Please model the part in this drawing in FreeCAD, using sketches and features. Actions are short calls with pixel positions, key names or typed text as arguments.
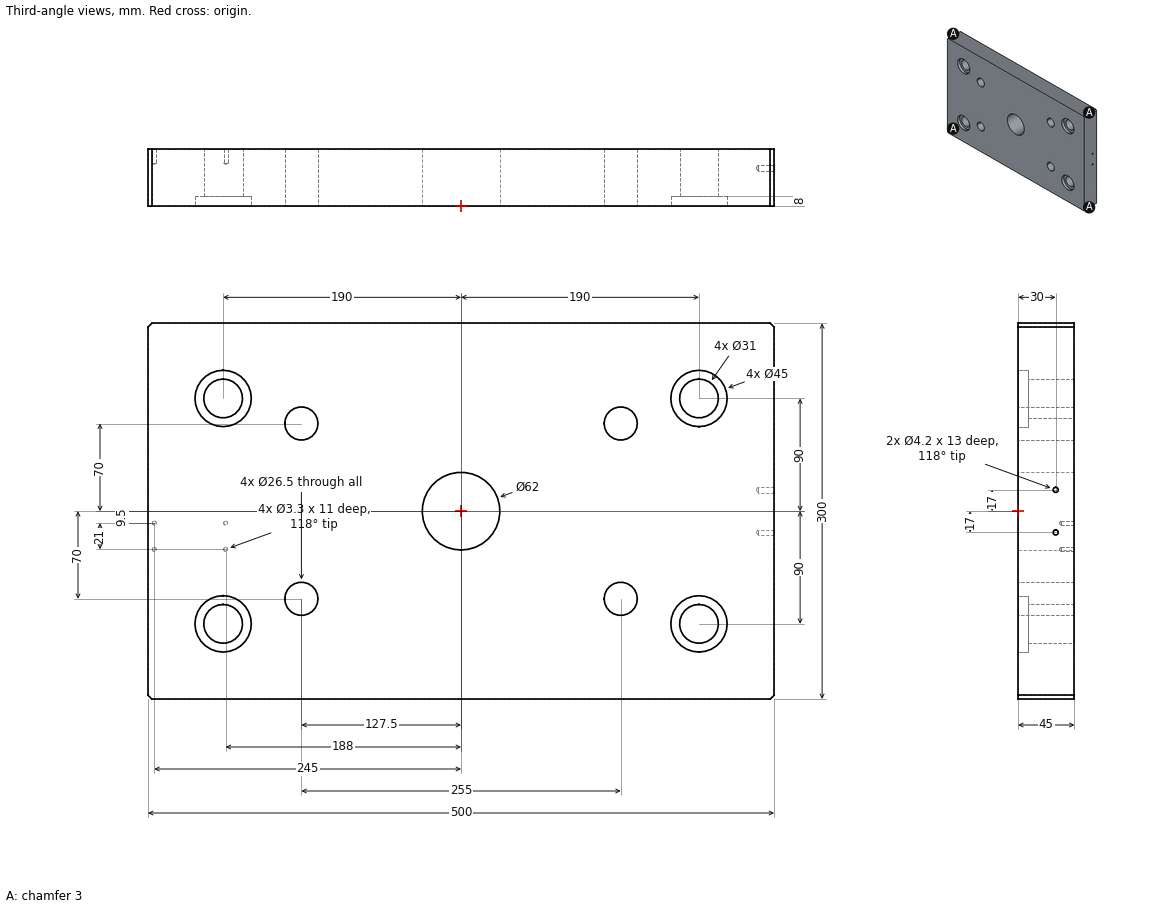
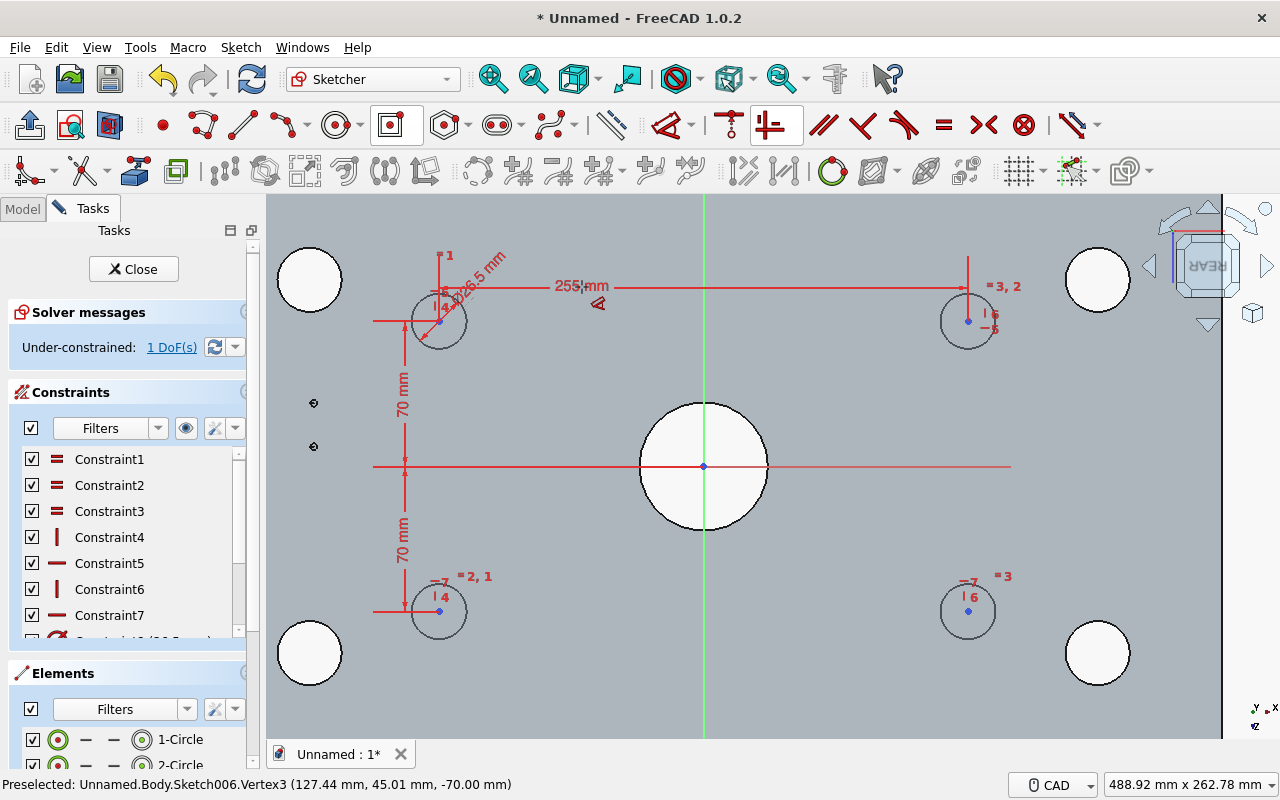
click(439, 321)
click(664, 287)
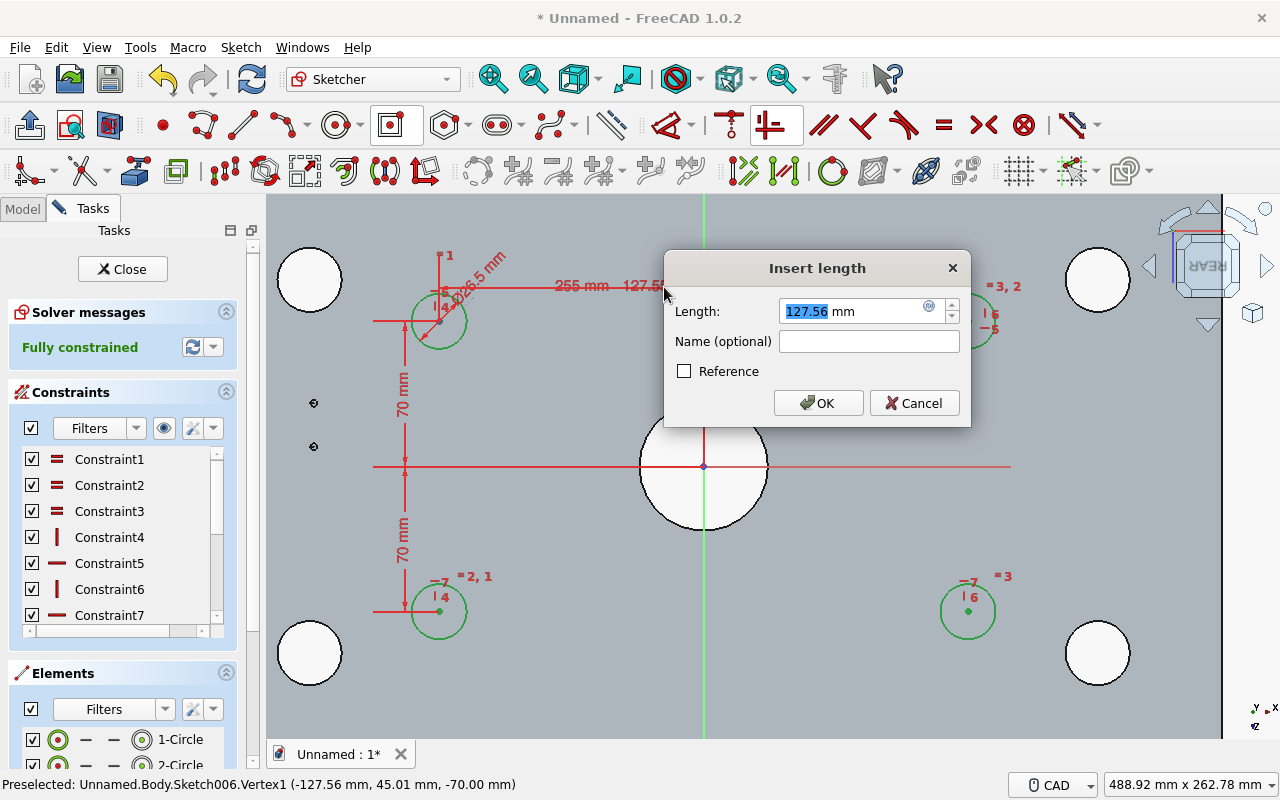
text(127.5)
key(Return)
key(Escape)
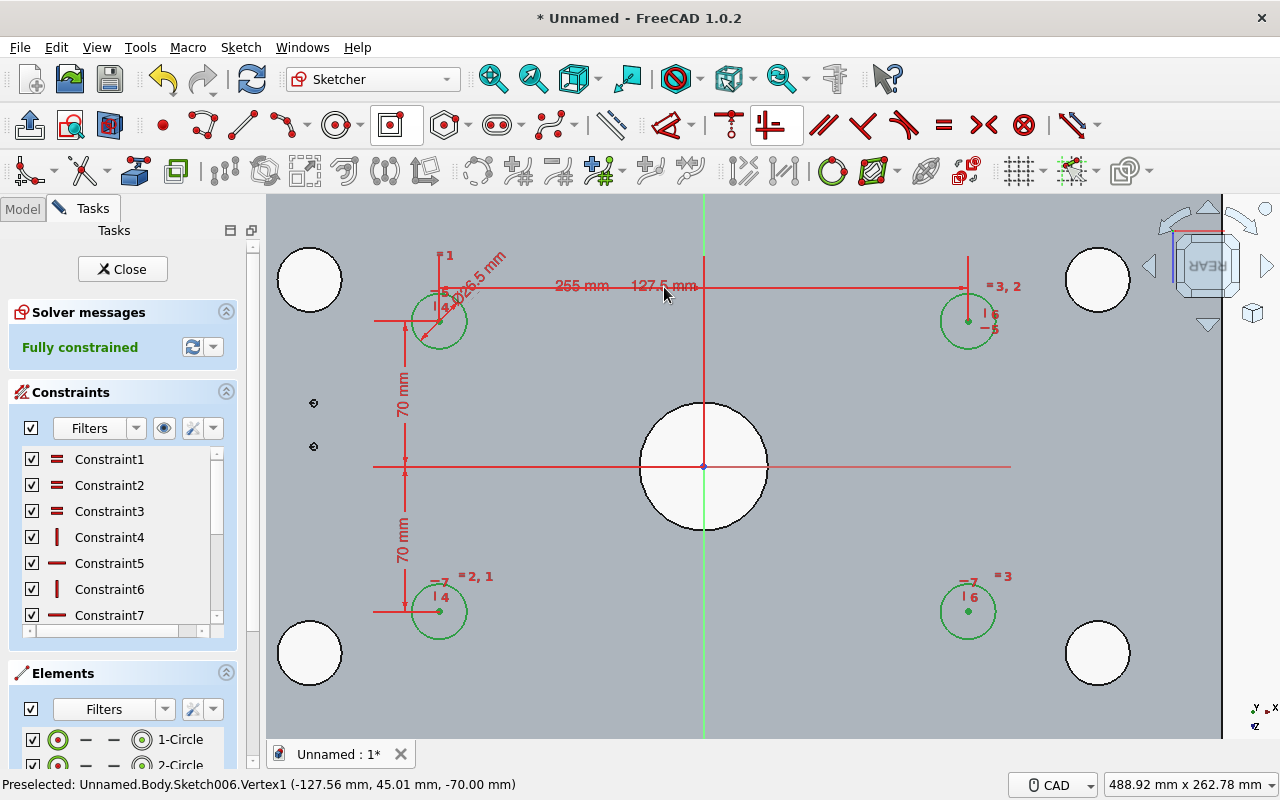
click(123, 269)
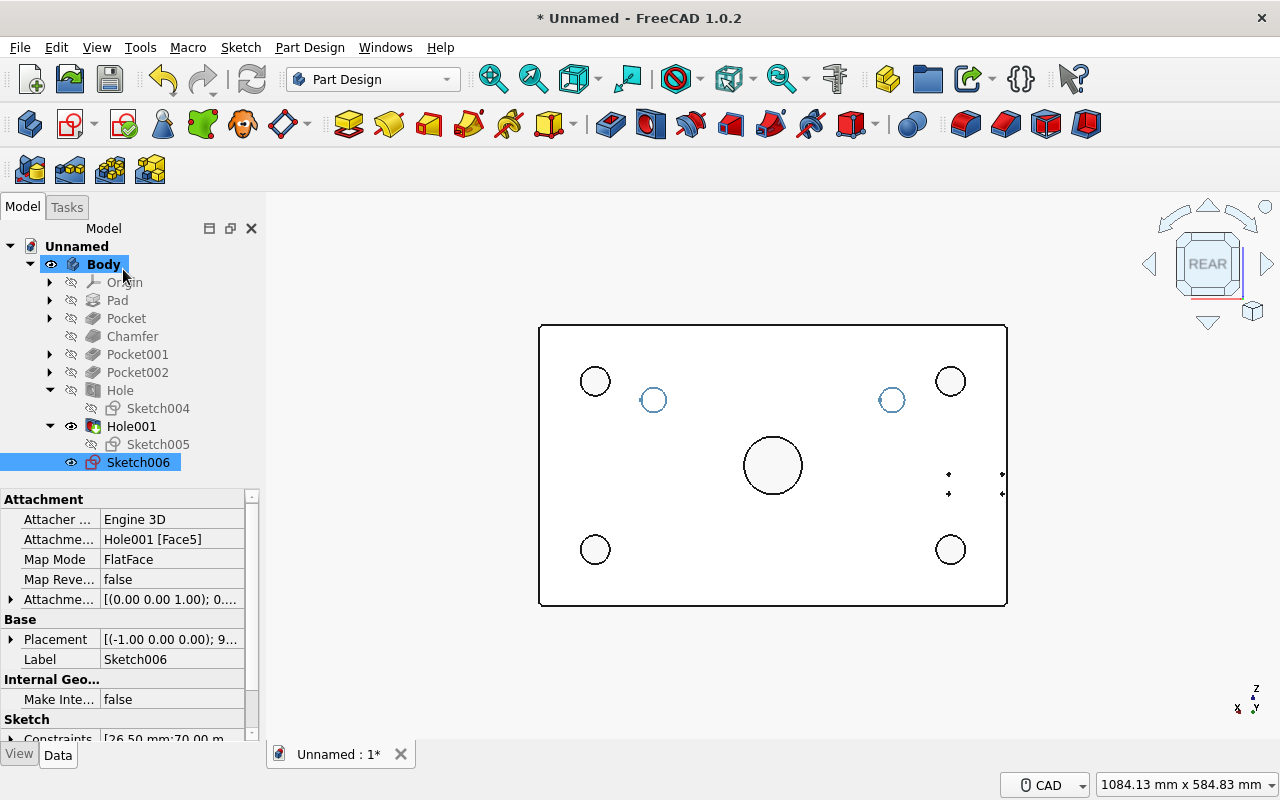
click(652, 124)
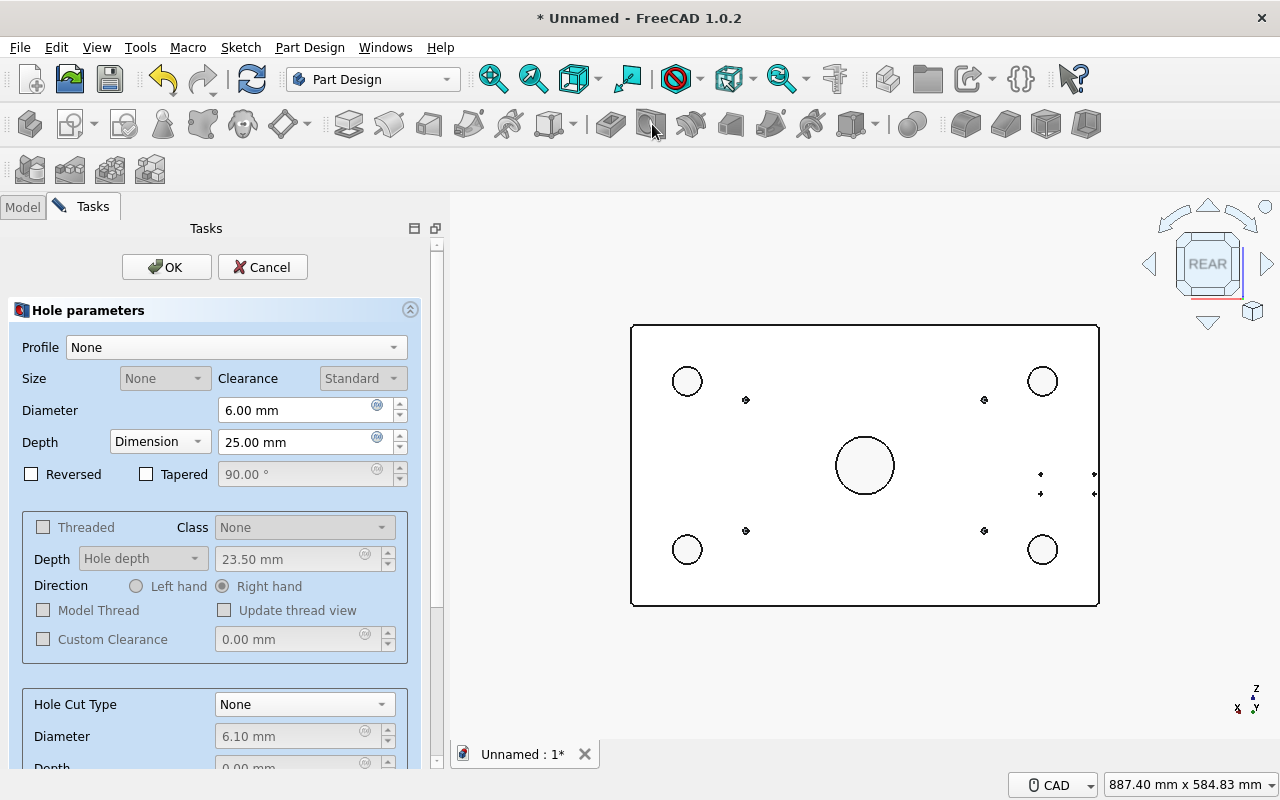
triple_click(305, 410)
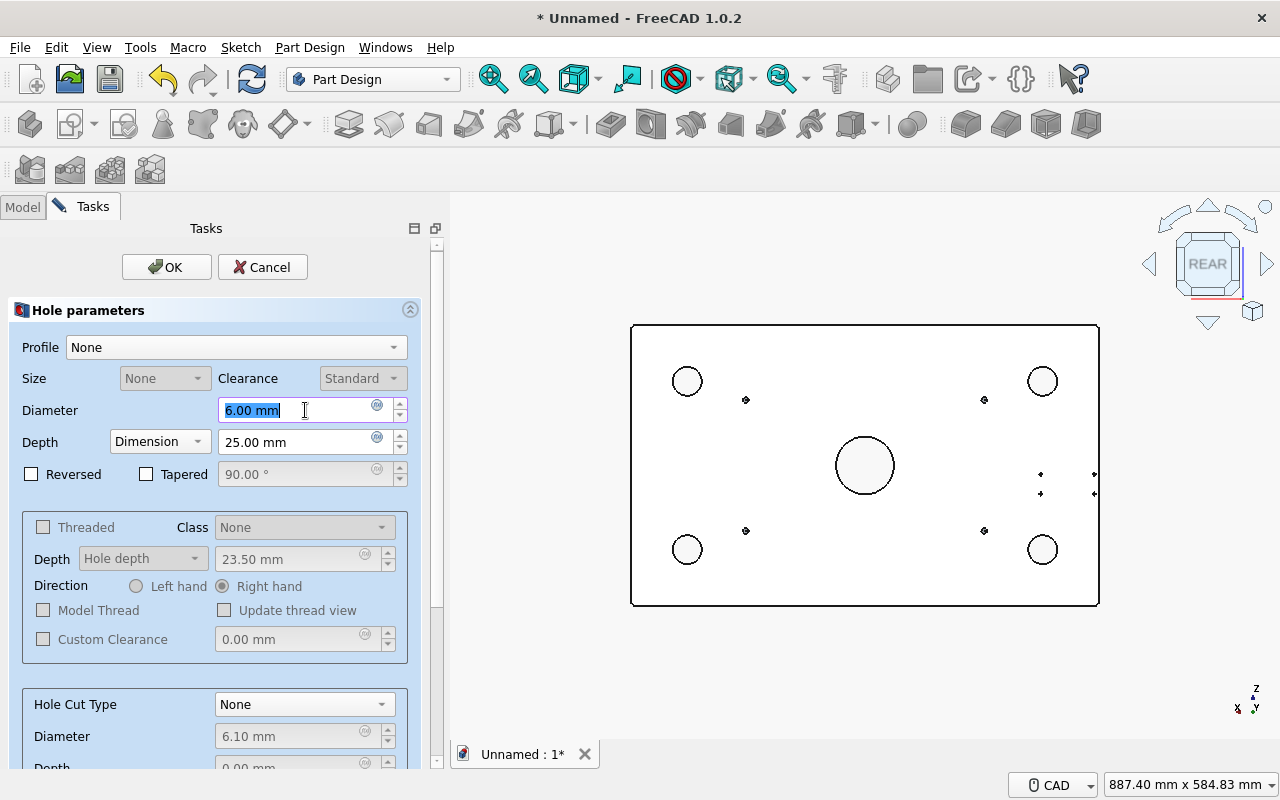
text(26.5)
key(Tab)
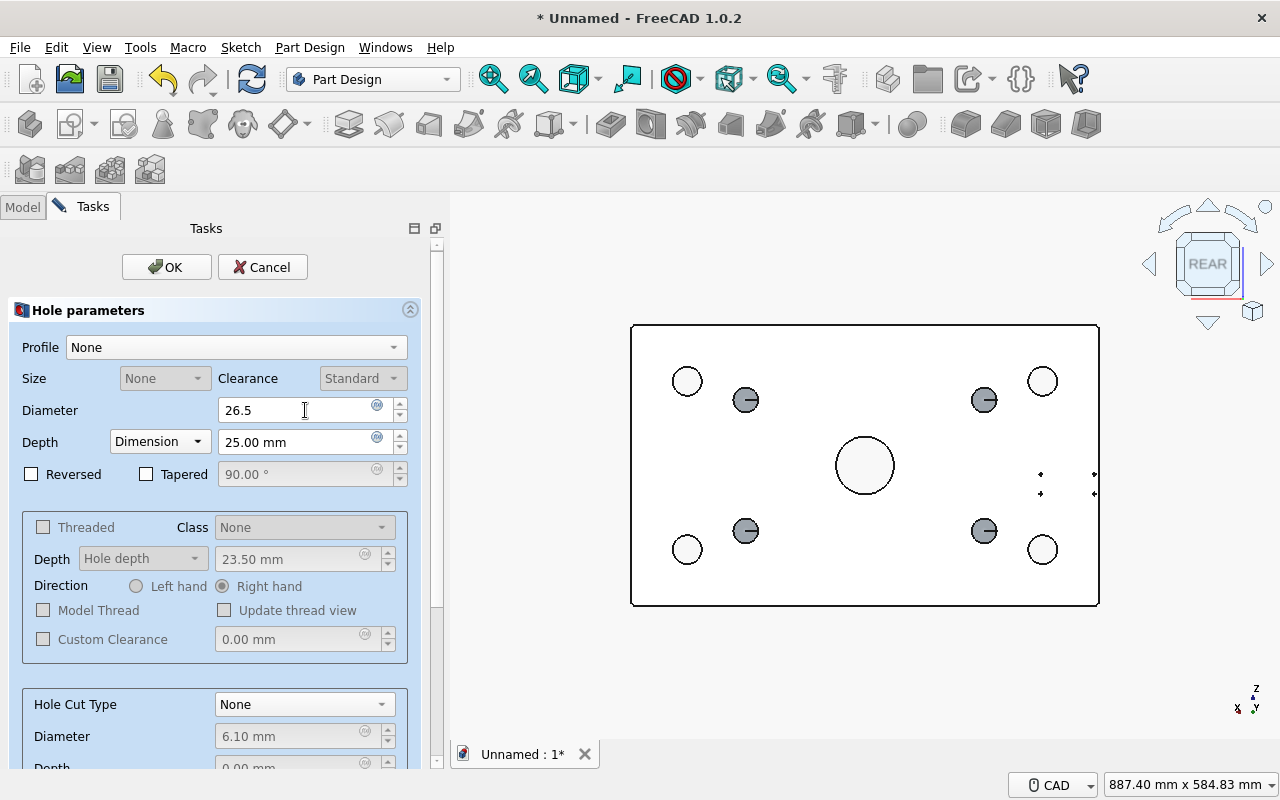
click(161, 442)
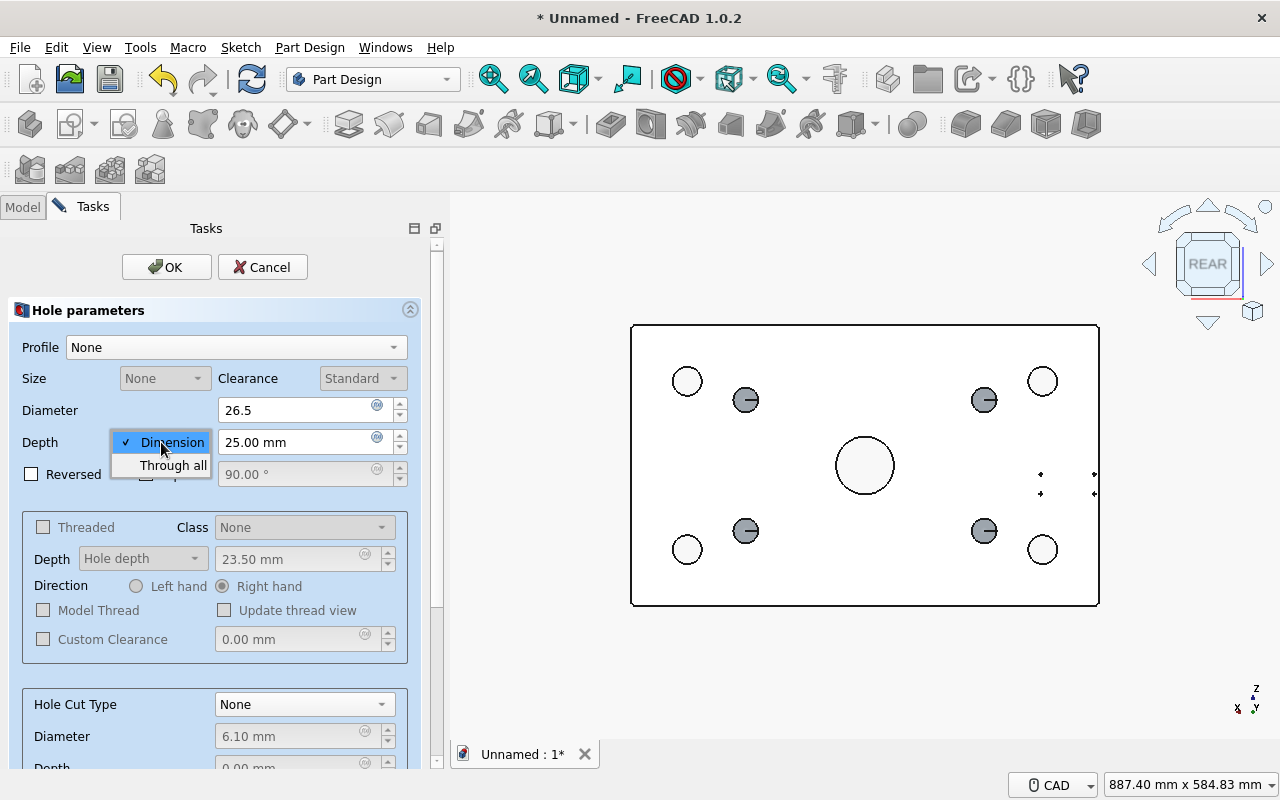
click(160, 466)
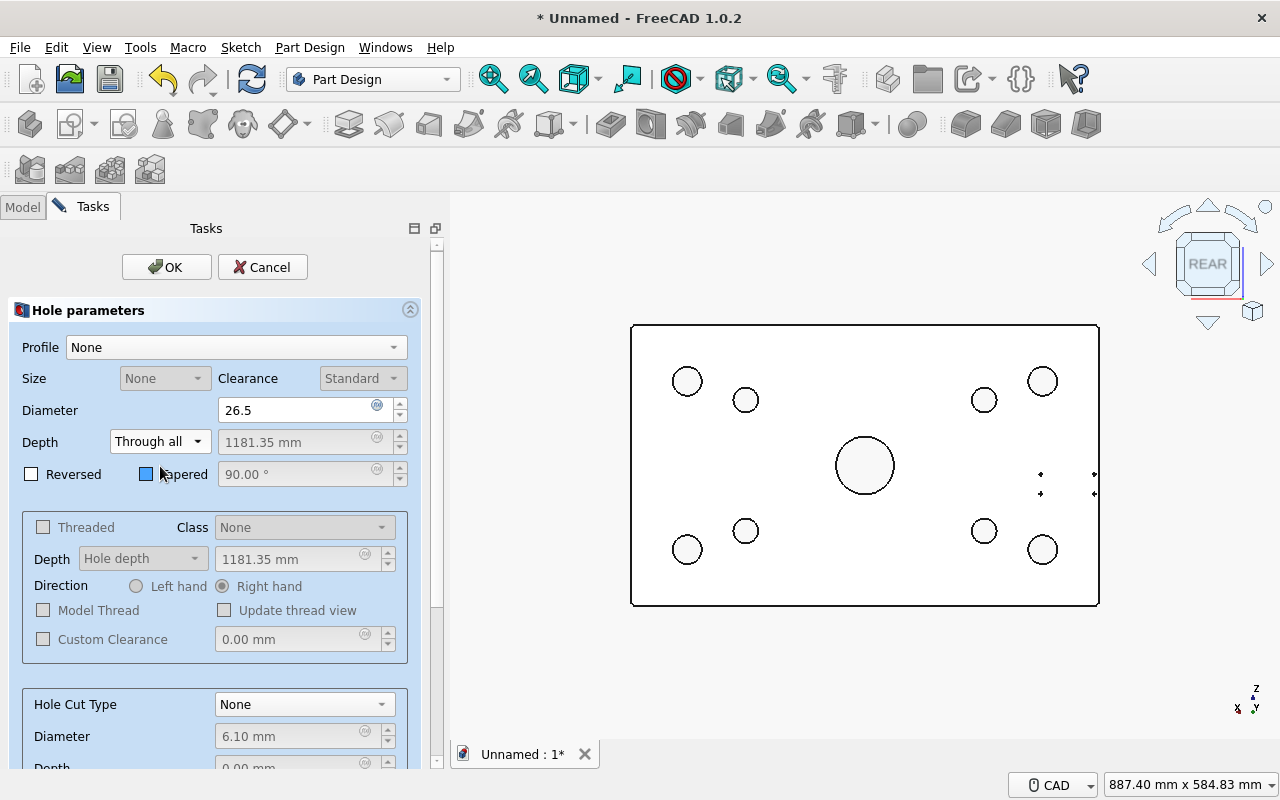
click(167, 267)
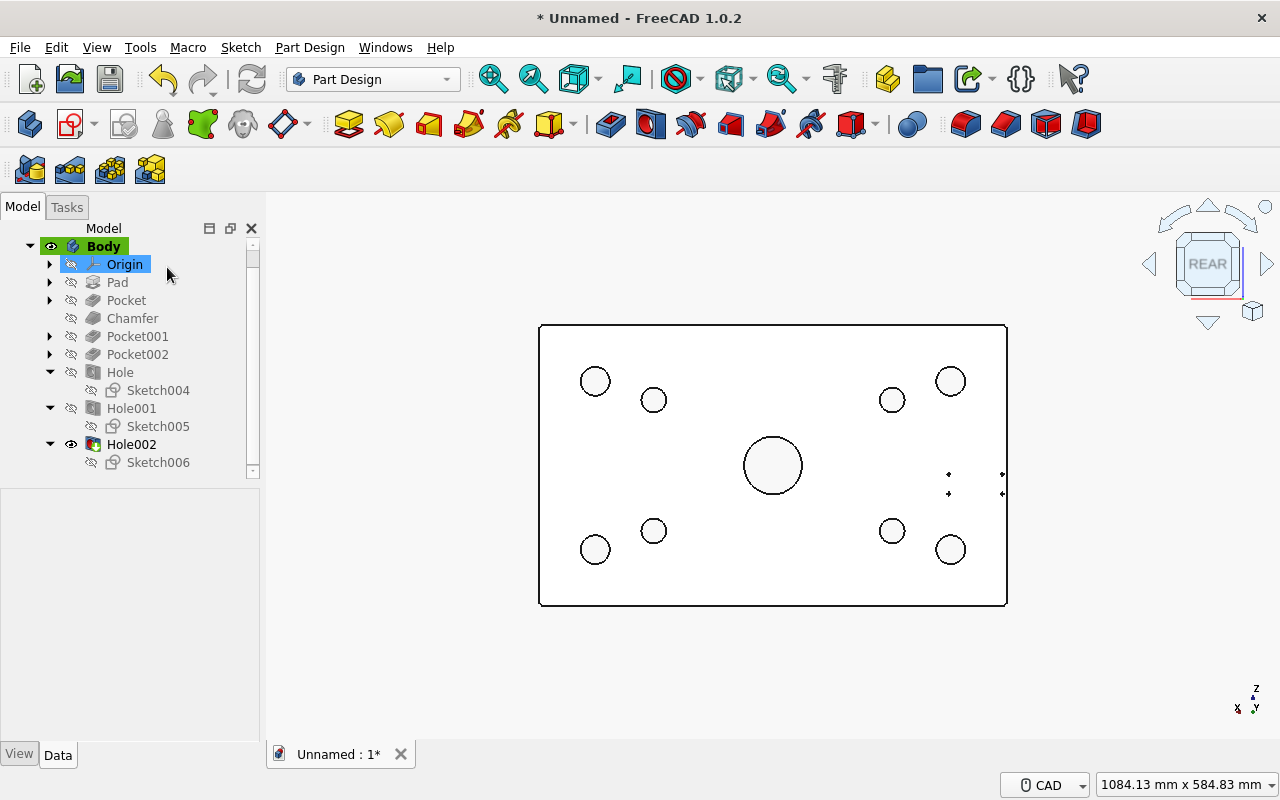
key(0)